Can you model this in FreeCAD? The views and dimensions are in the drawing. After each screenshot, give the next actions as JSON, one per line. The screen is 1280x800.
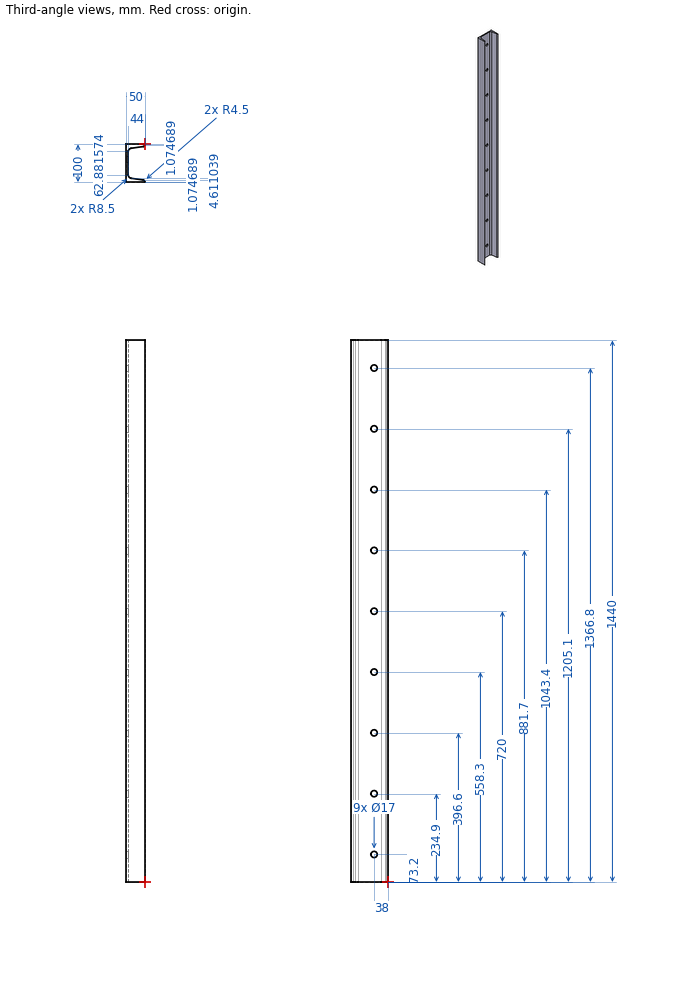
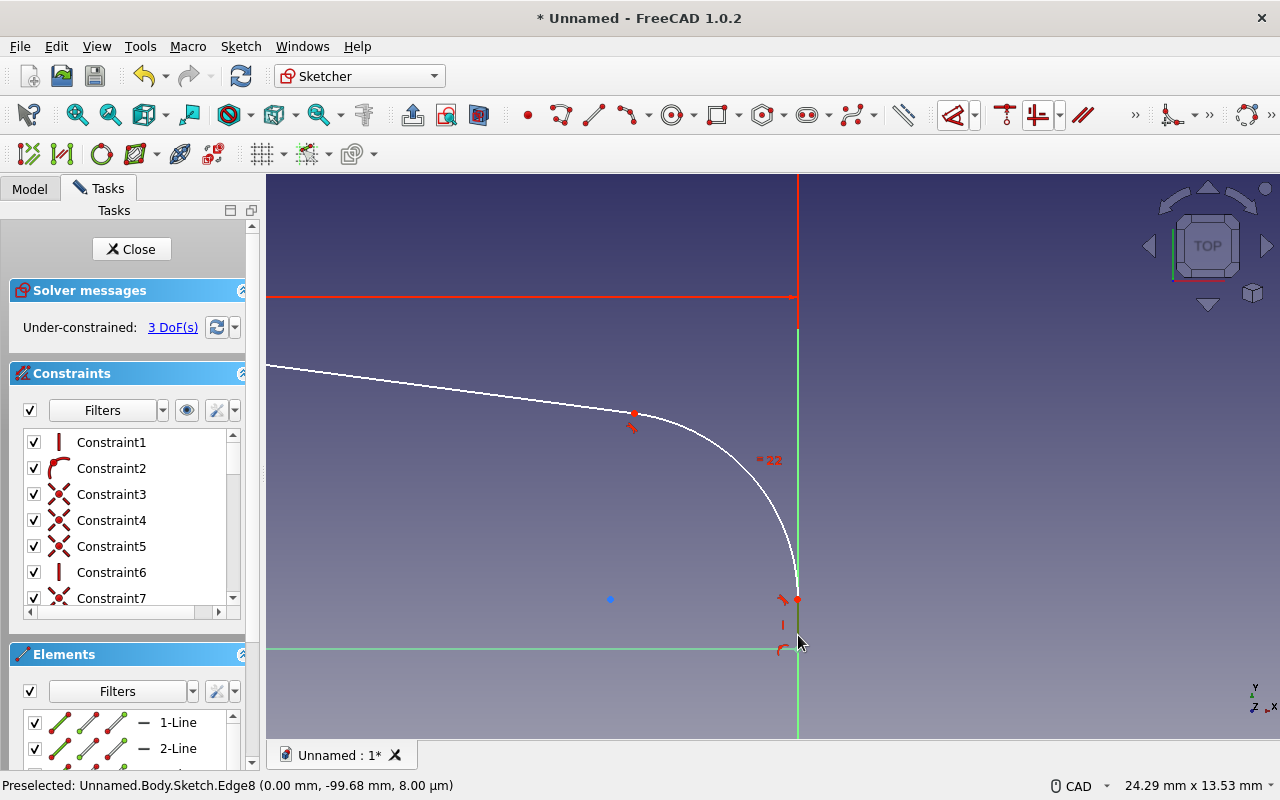
{"action": "left_click", "coordinate": [974, 116]}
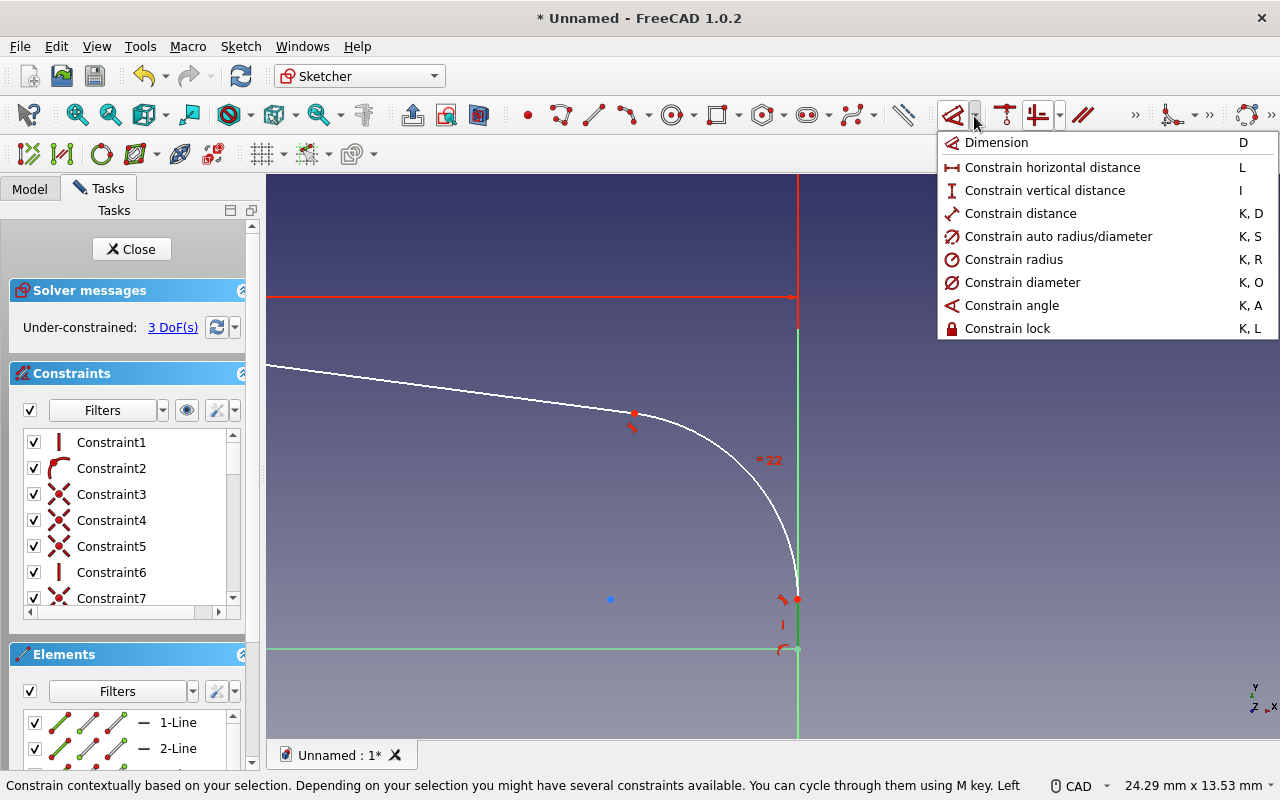
{"action": "left_click", "coordinate": [1108, 190]}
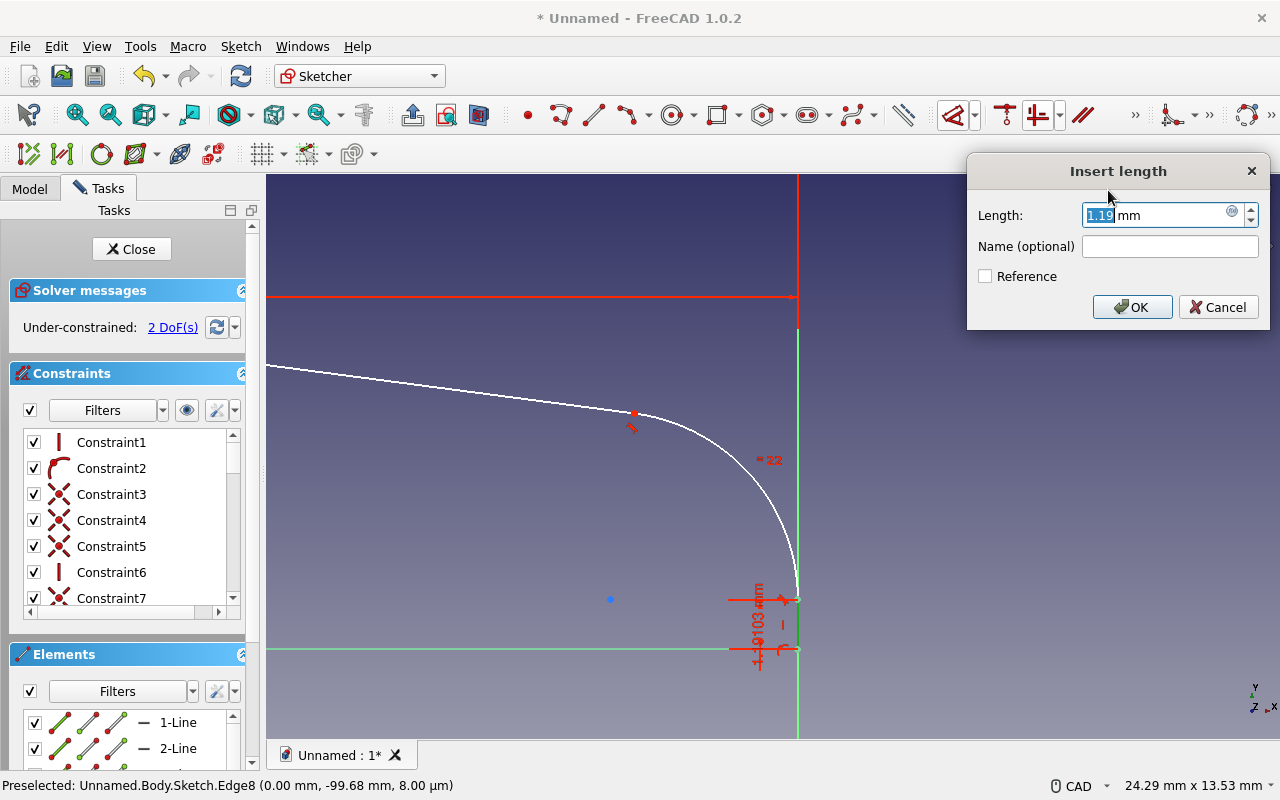
{"action": "type", "text": "1.074689"}
{"action": "key", "text": "Return"}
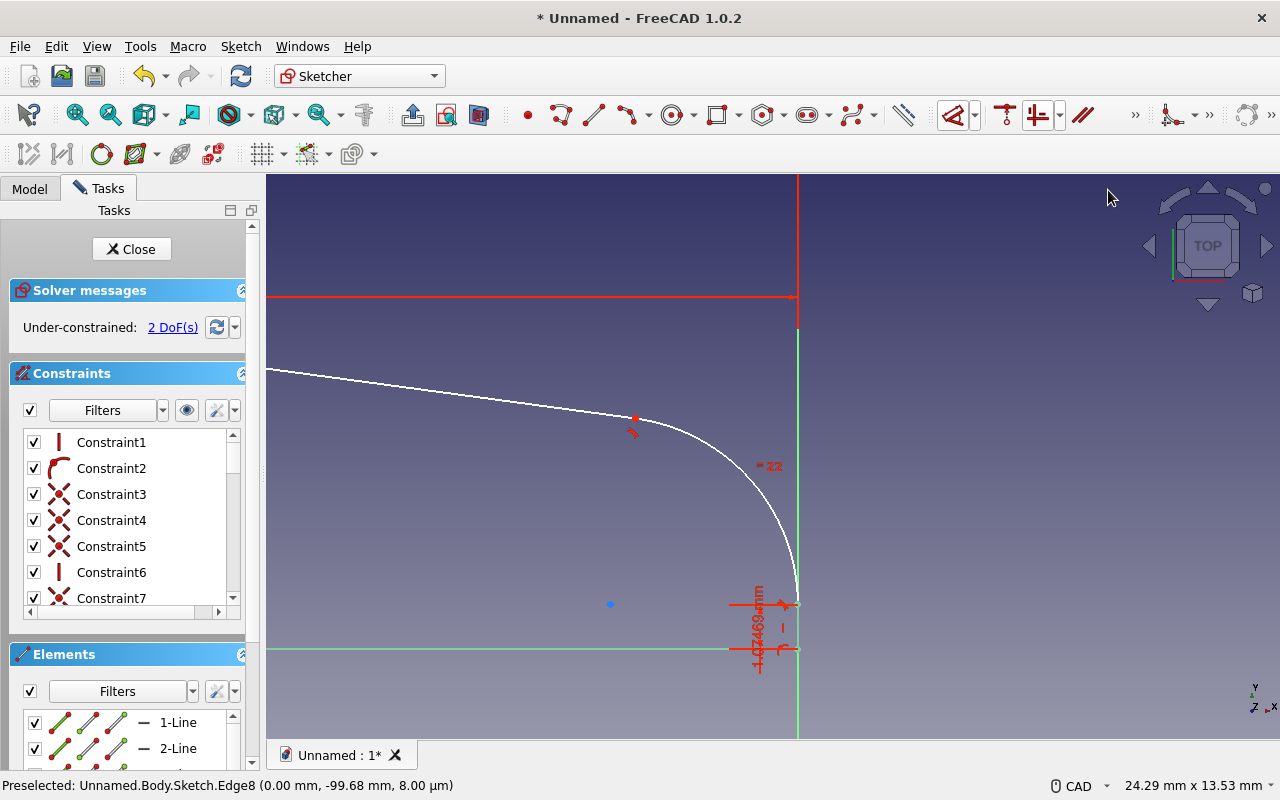
{"action": "scroll", "coordinate": [799, 646], "scroll_direction": "down", "scroll_amount": 12}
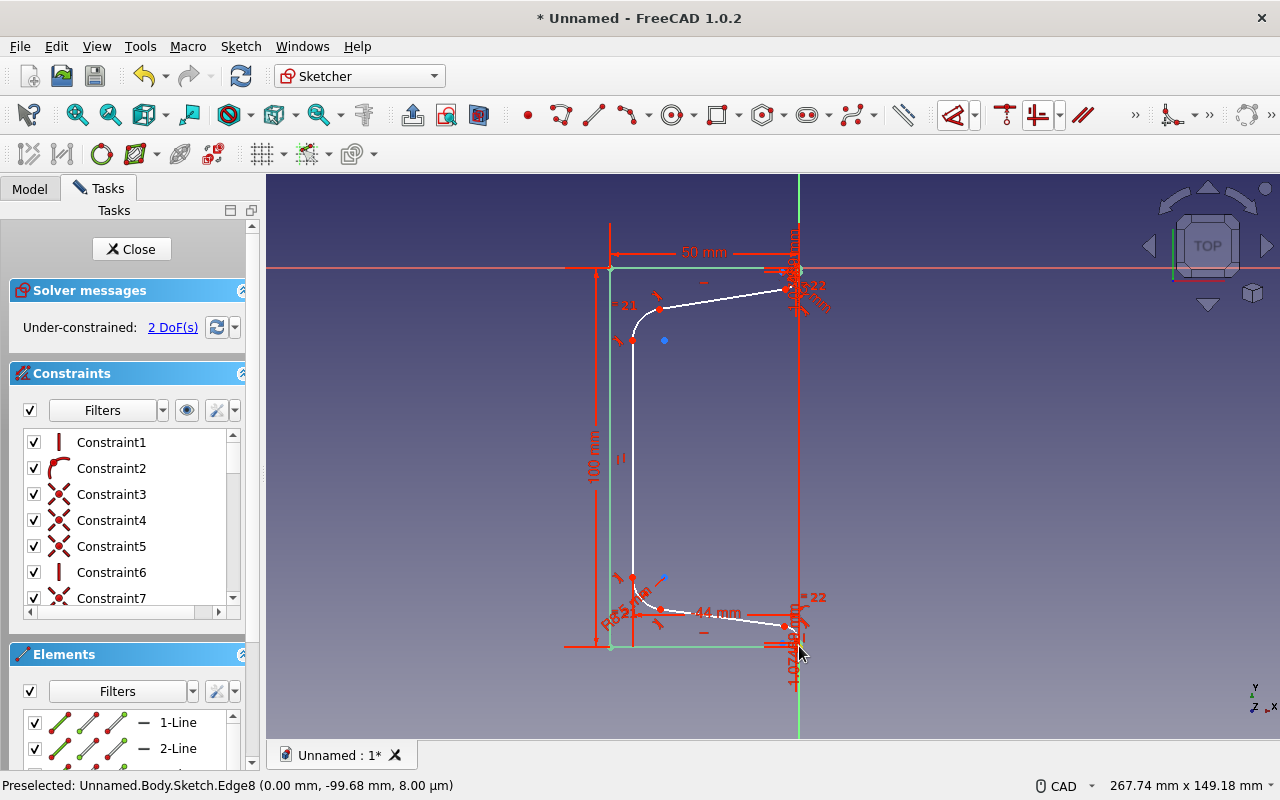
{"action": "left_click", "coordinate": [633, 506]}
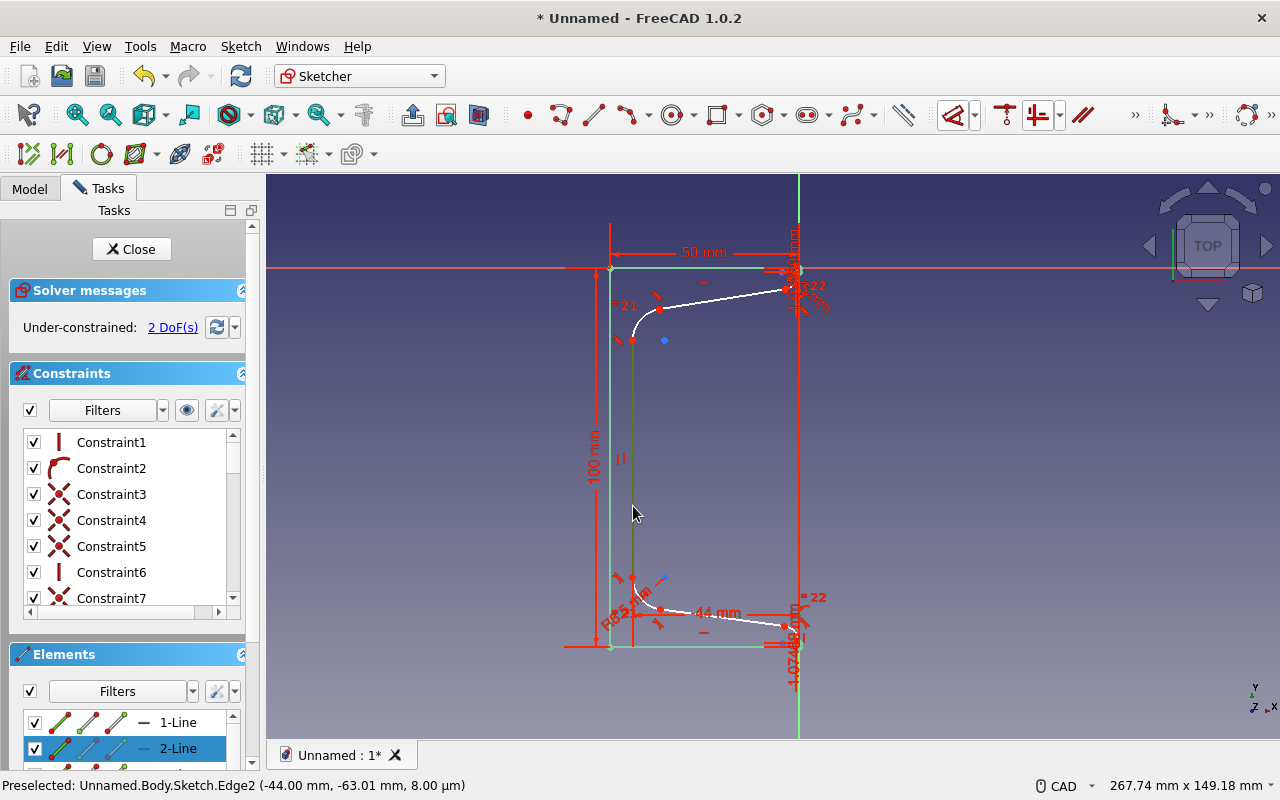
{"action": "left_click", "coordinate": [974, 116]}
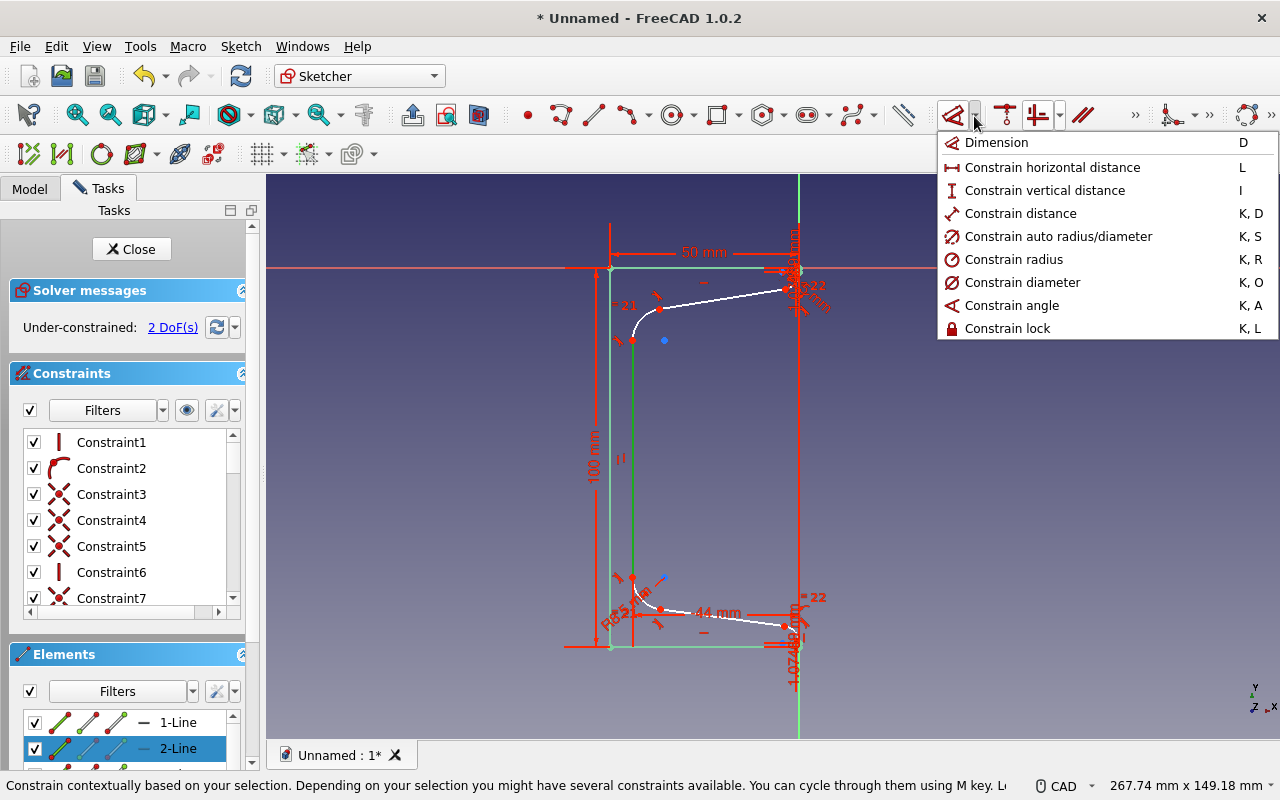
{"action": "left_click", "coordinate": [1108, 190]}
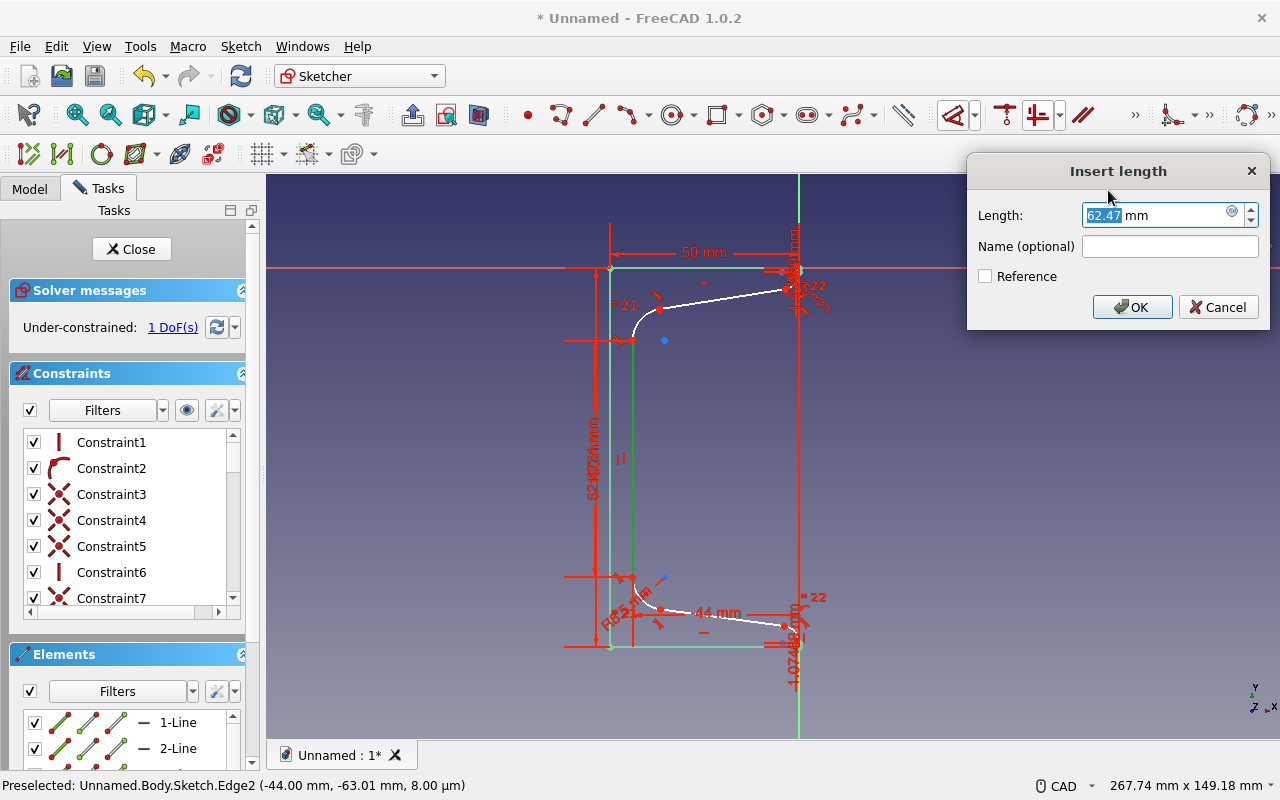
{"action": "type", "text": "62.881574"}
{"action": "key", "text": "Return"}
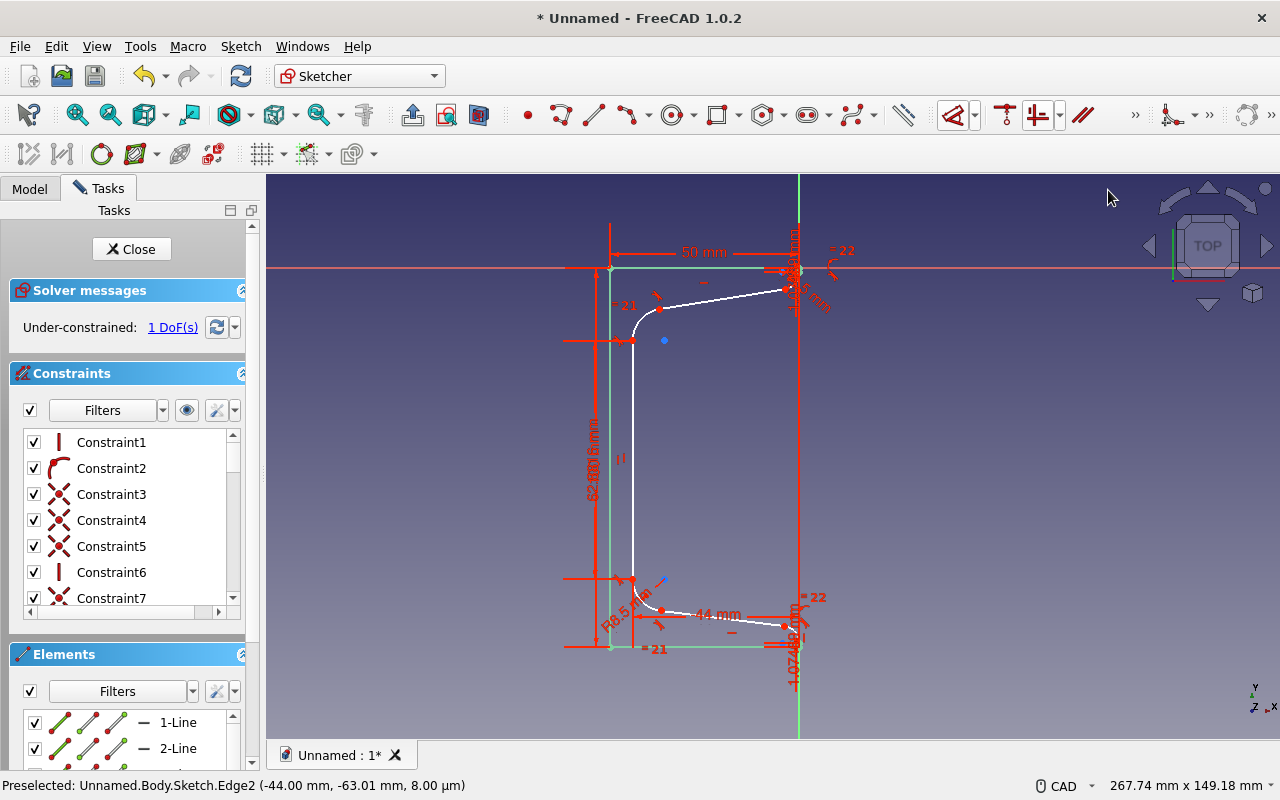
{"action": "scroll", "coordinate": [747, 622], "scroll_direction": "up", "scroll_amount": 5}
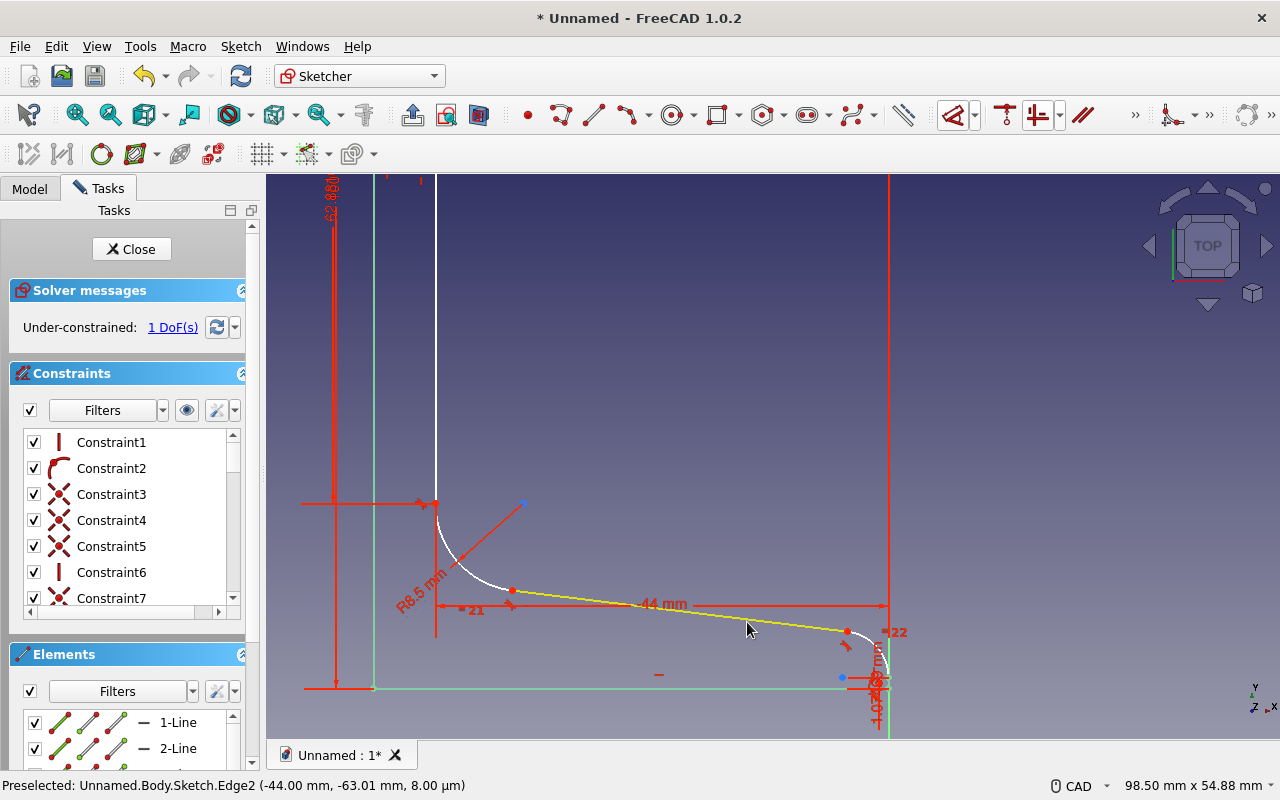
{"action": "left_click", "coordinate": [747, 619]}